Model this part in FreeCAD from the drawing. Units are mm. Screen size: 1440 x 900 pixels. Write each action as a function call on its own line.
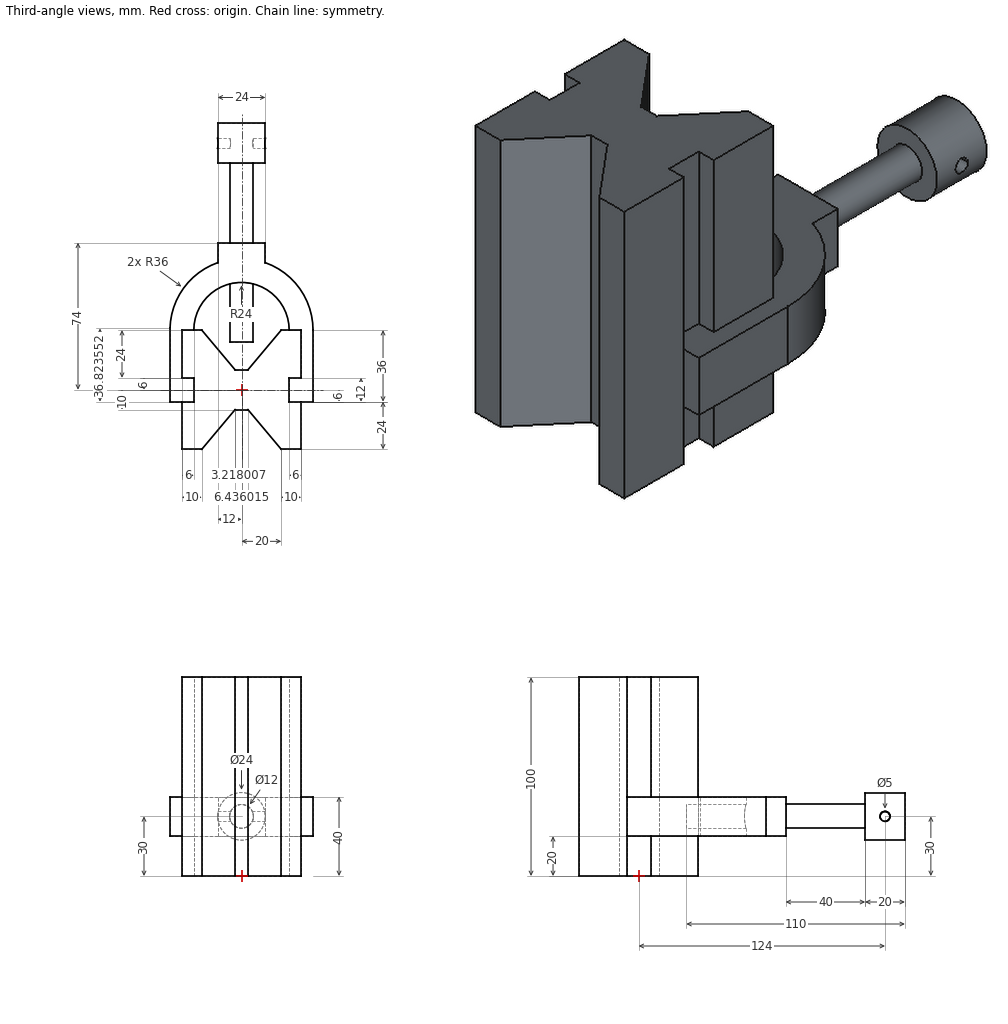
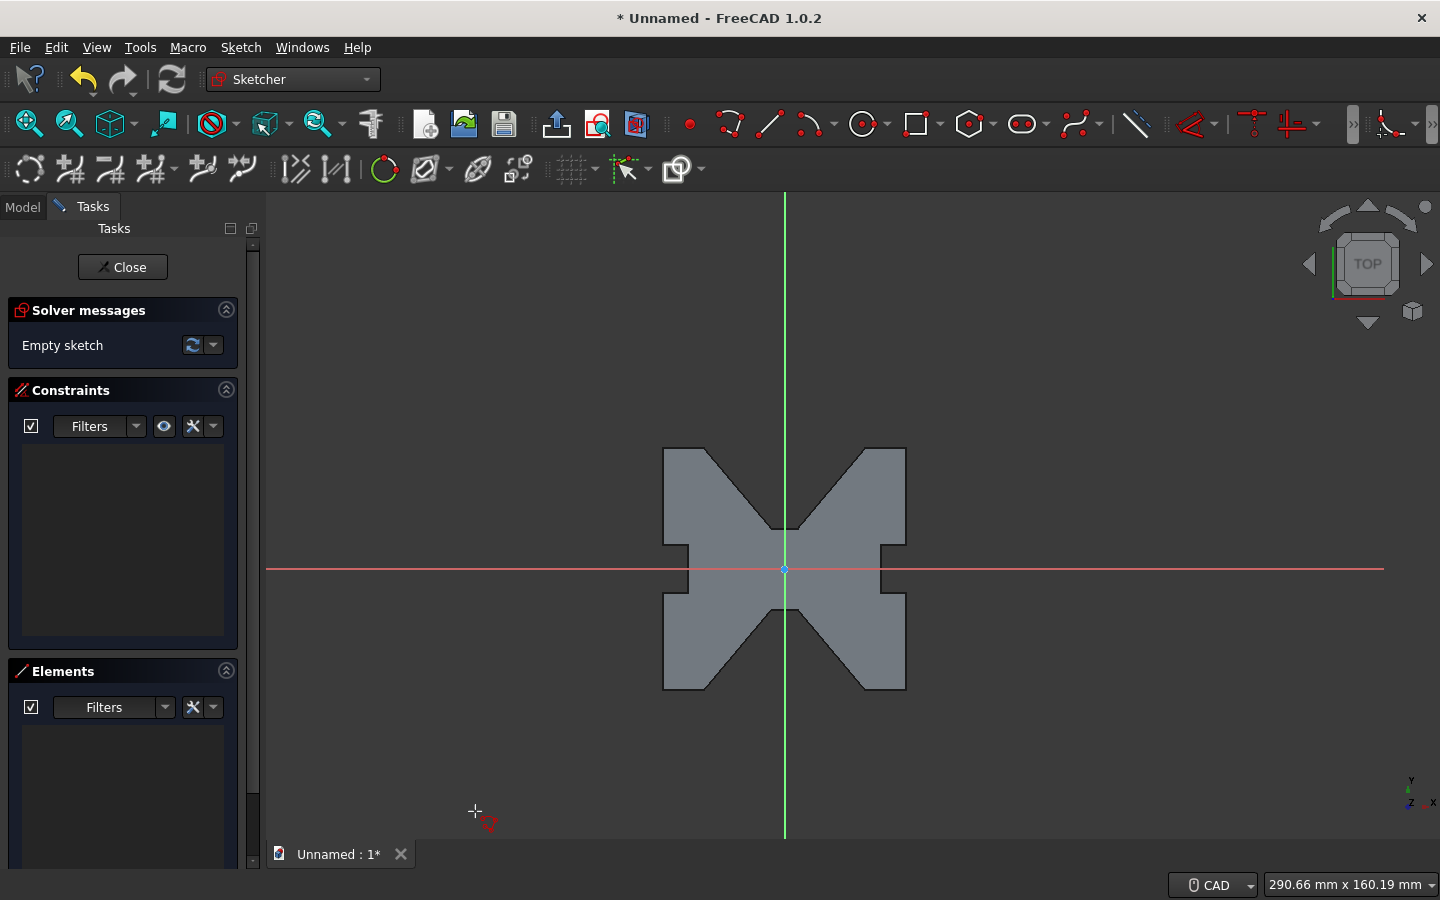
click(688, 448)
click(663, 448)
click(663, 545)
click(688, 545)
click(688, 593)
click(639, 593)
click(639, 445)
right_click(639, 445)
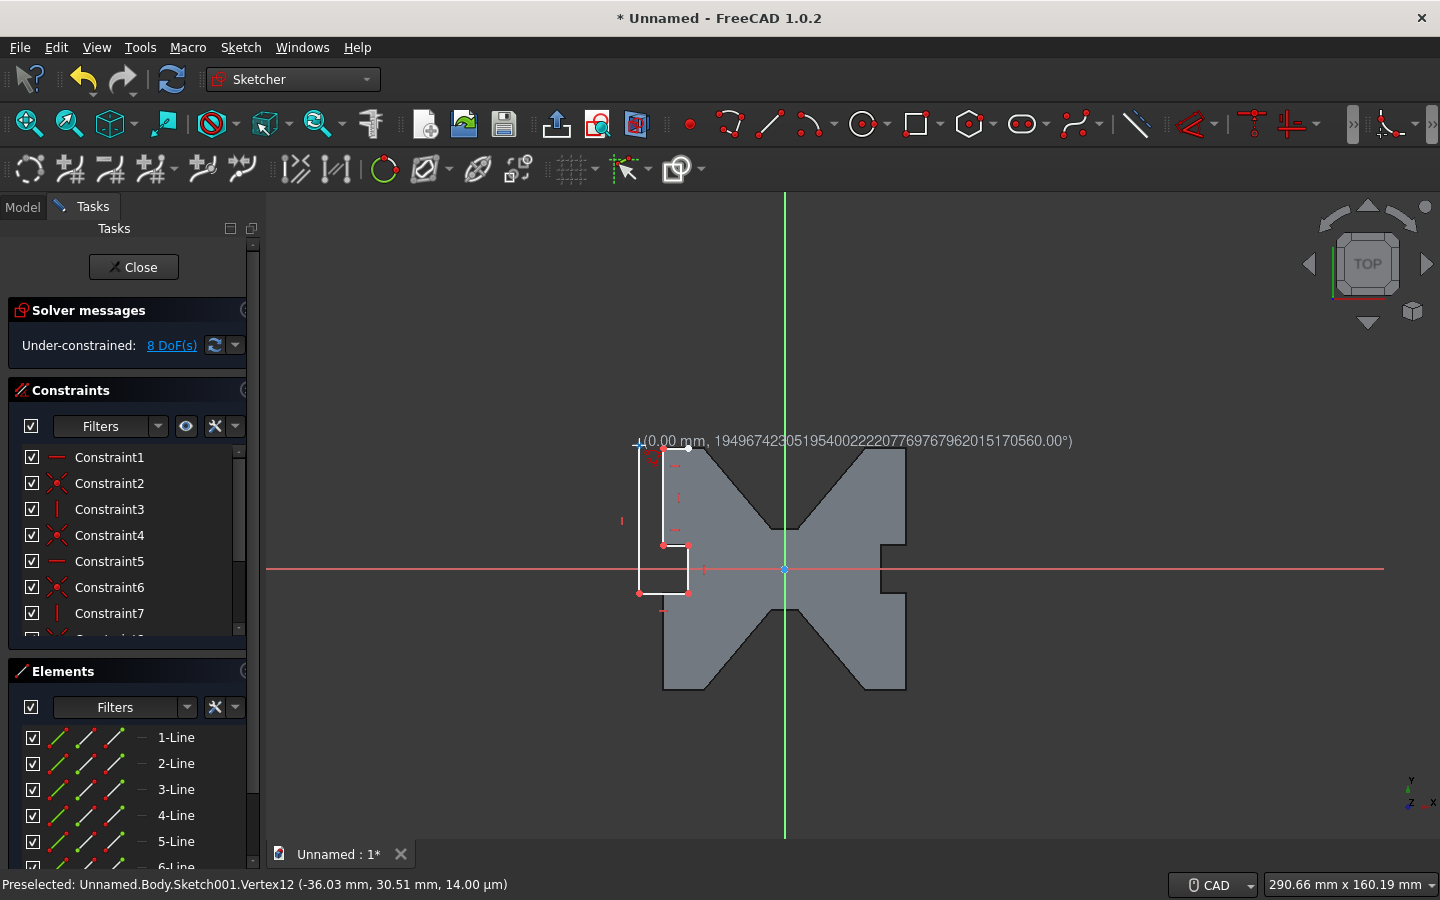
click(736, 311)
click(736, 270)
click(833, 270)
click(833, 311)
right_click(833, 311)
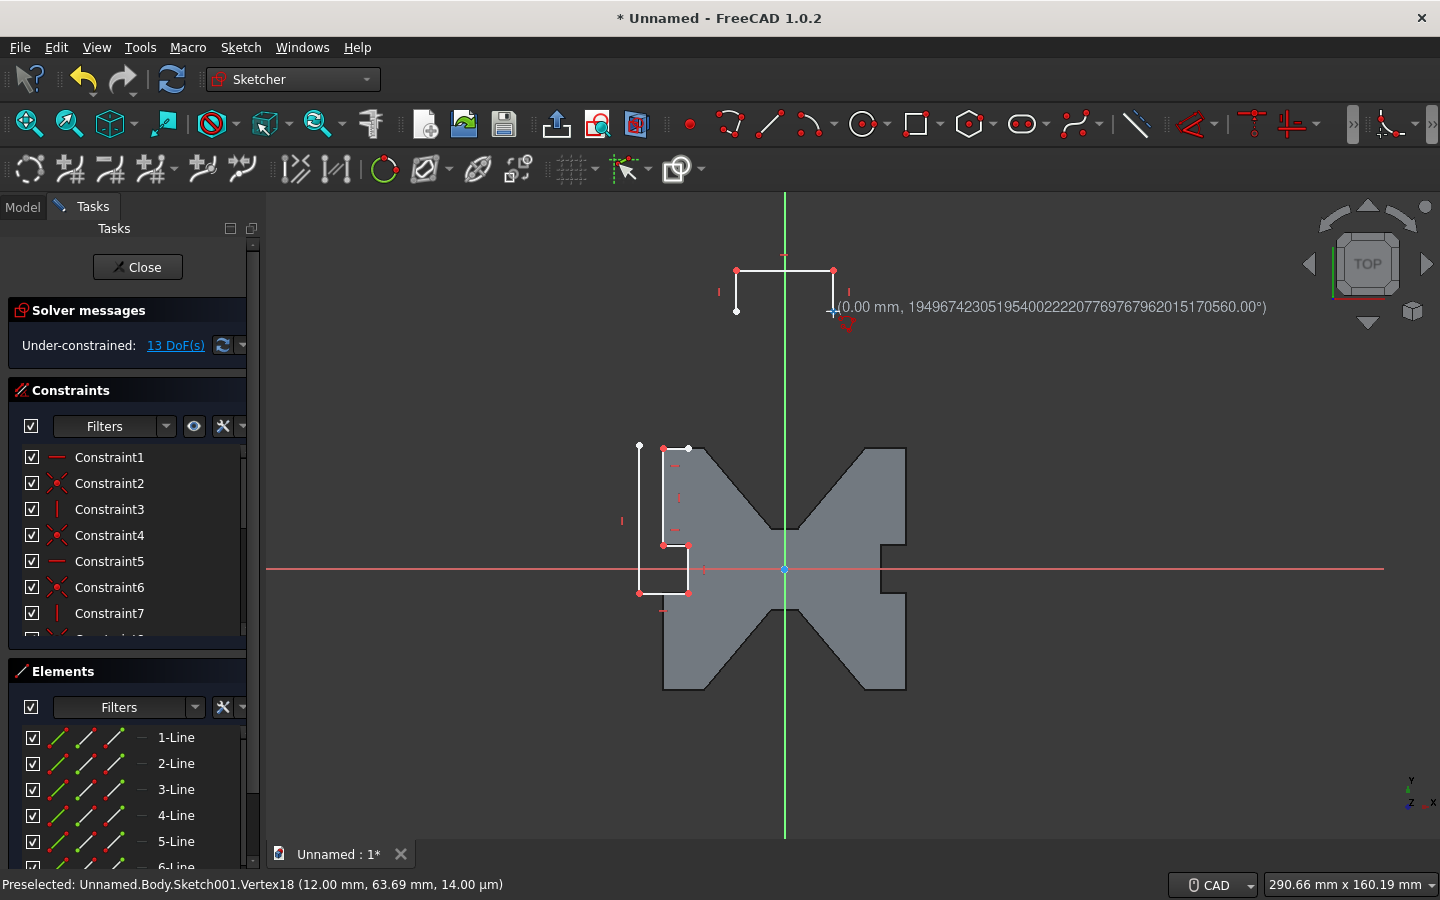
click(930, 448)
click(930, 593)
click(881, 593)
click(881, 545)
click(906, 545)
click(906, 448)
click(881, 448)
right_click(881, 448)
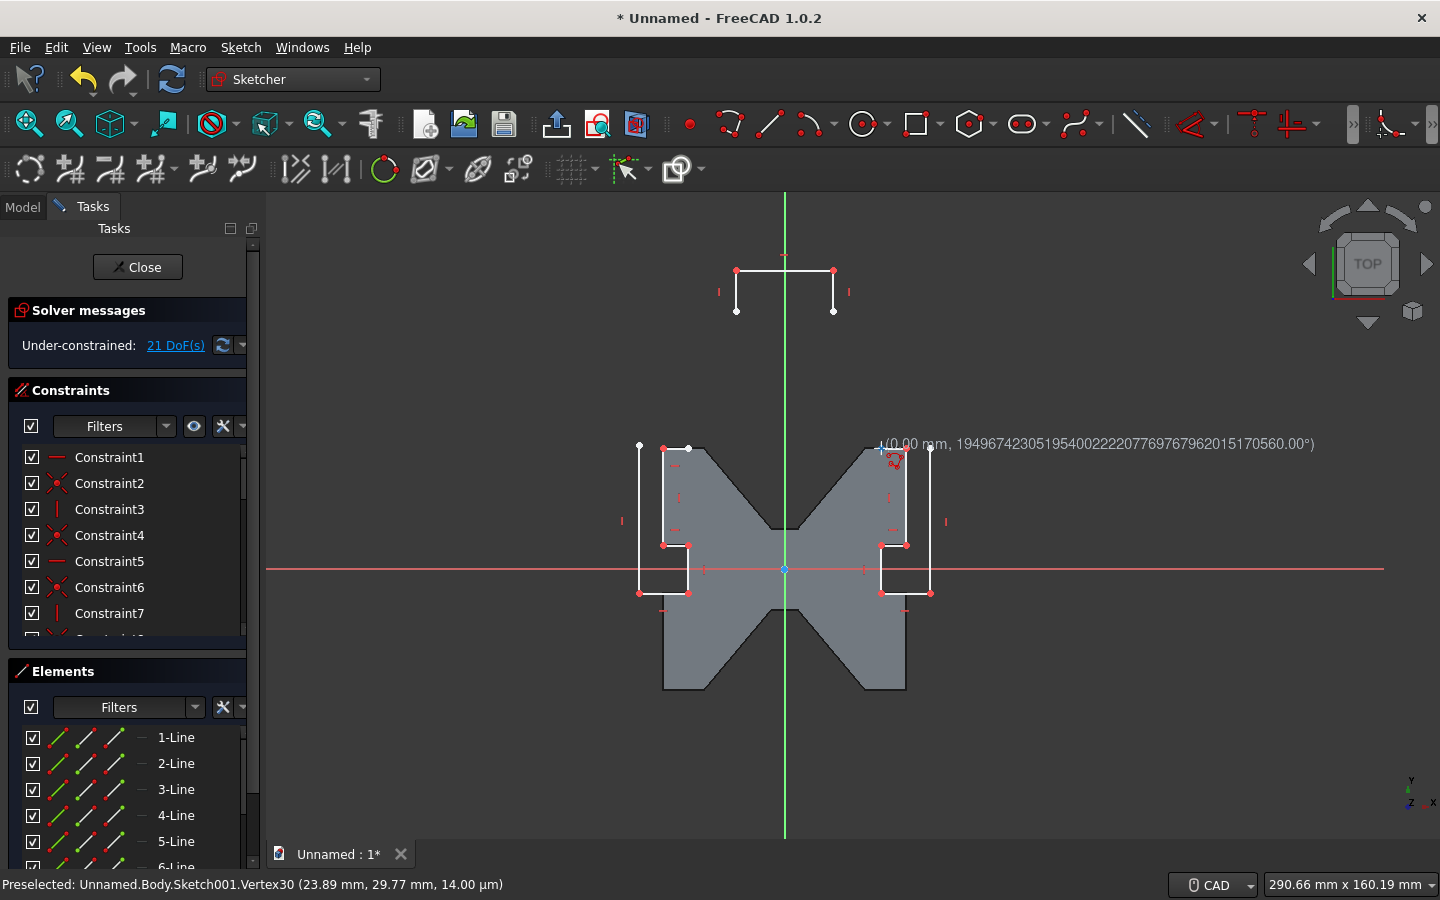
key(g)
key(3)
key(a)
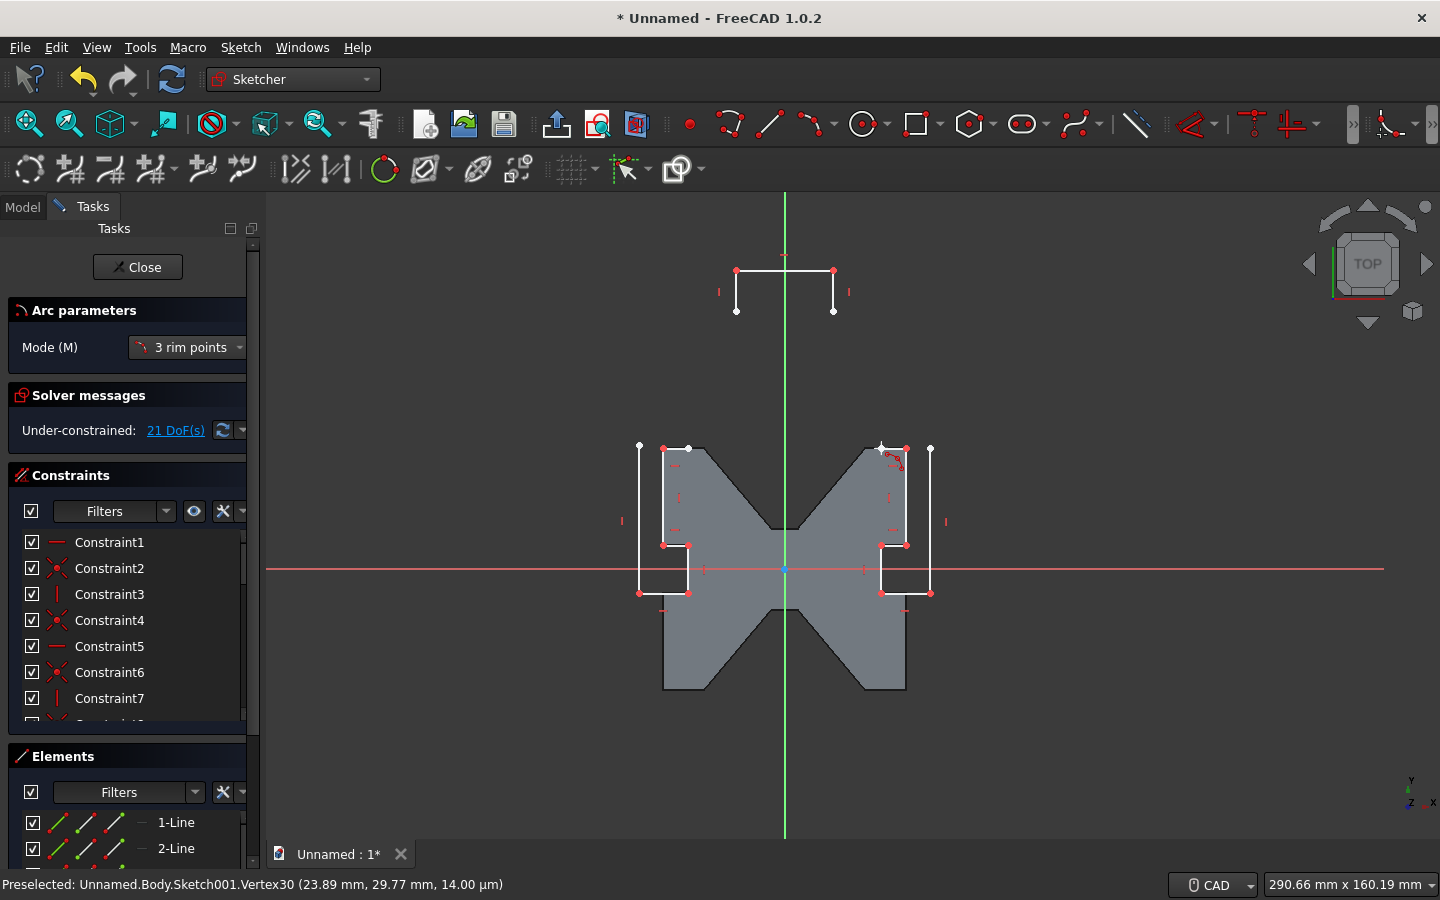
click(639, 446)
click(736, 312)
click(667, 363)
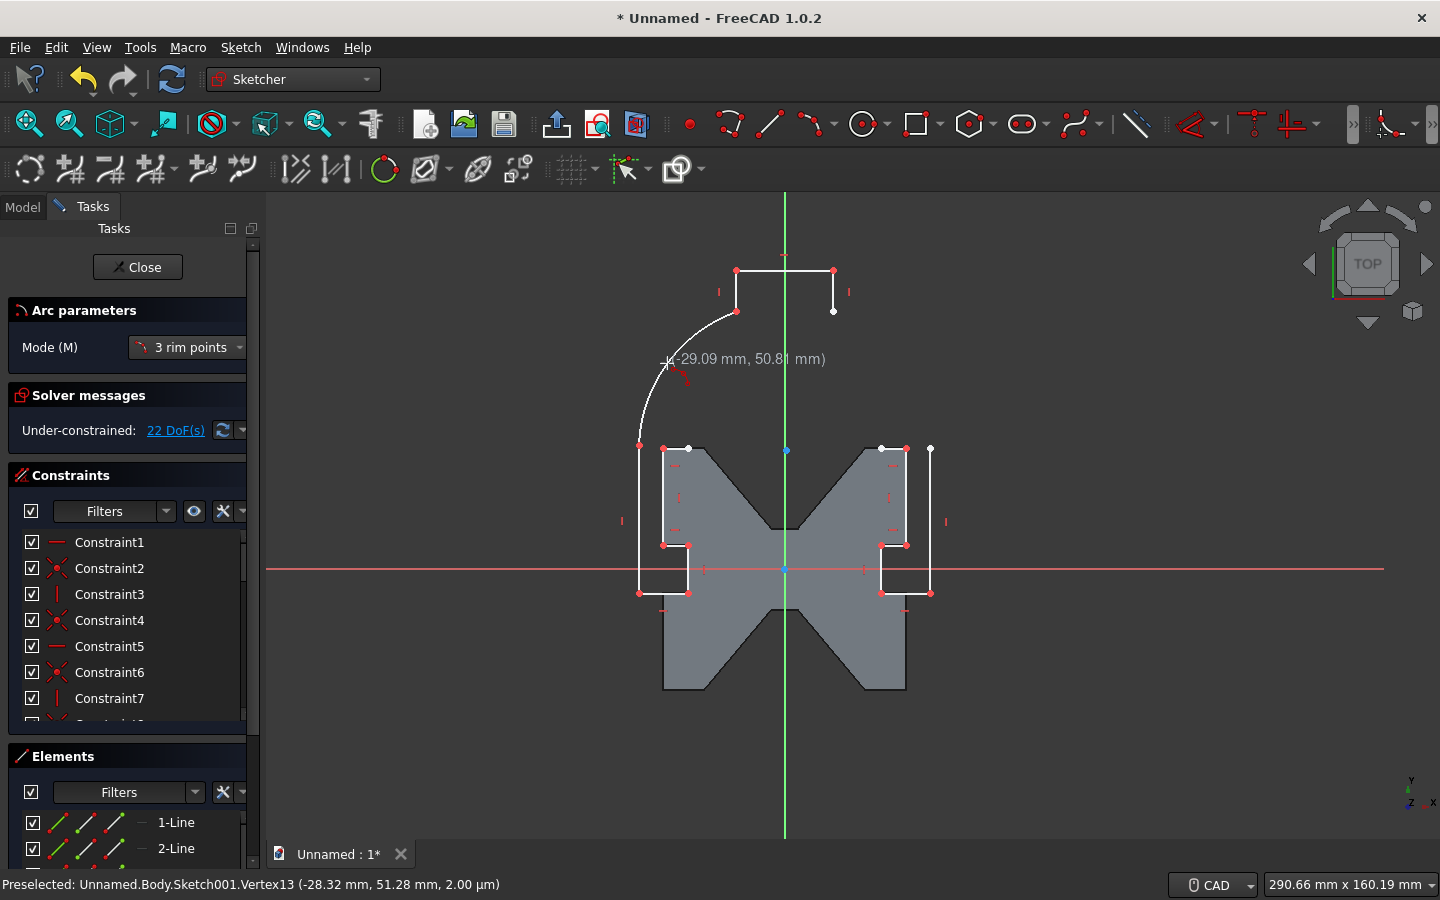
click(833, 312)
click(930, 449)
click(903, 364)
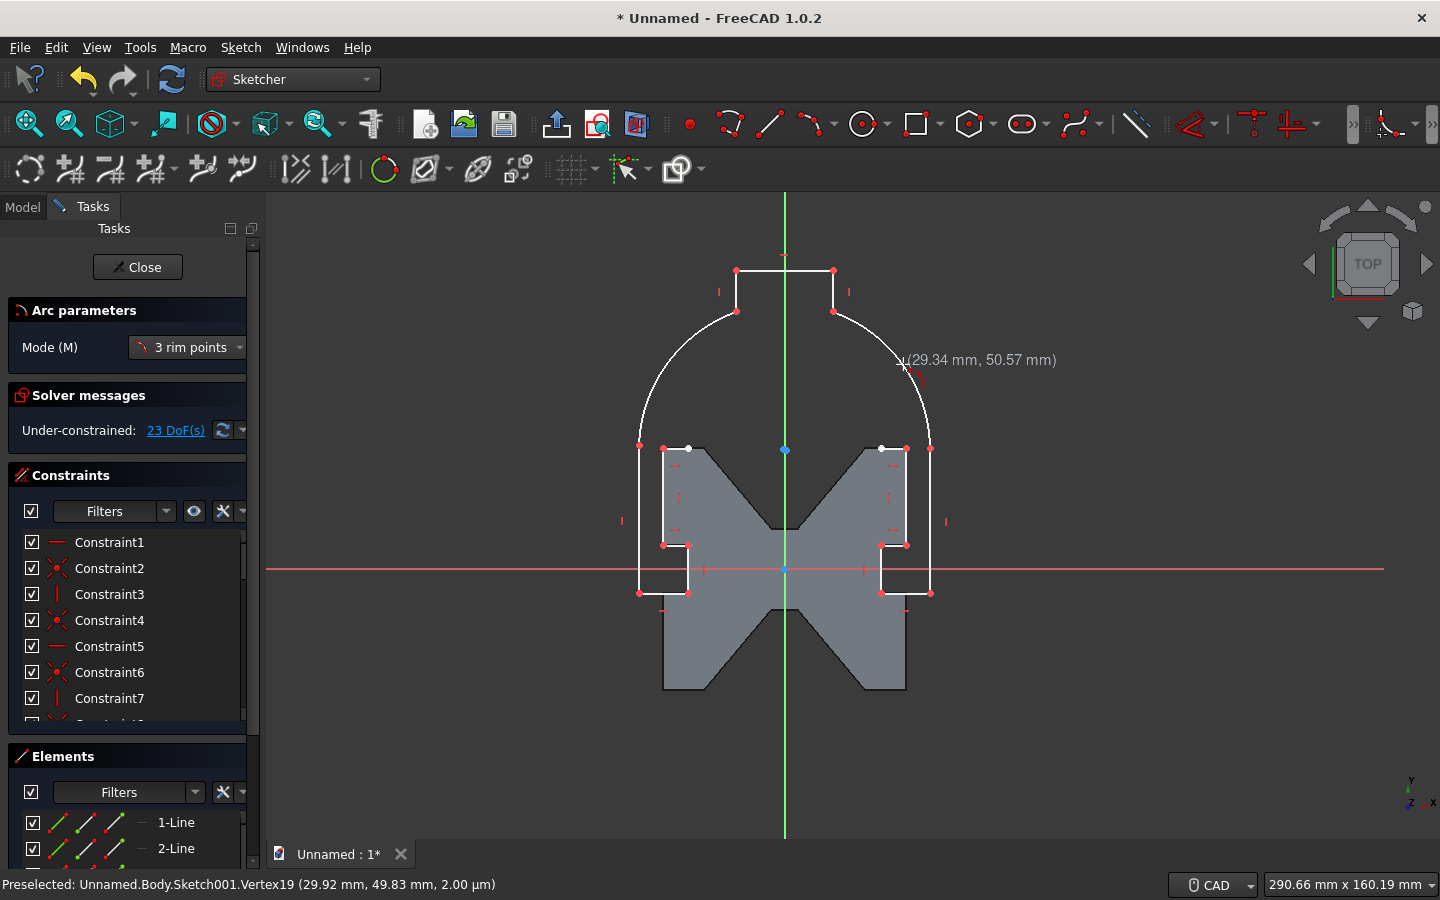
scroll(881, 448, up, 2)